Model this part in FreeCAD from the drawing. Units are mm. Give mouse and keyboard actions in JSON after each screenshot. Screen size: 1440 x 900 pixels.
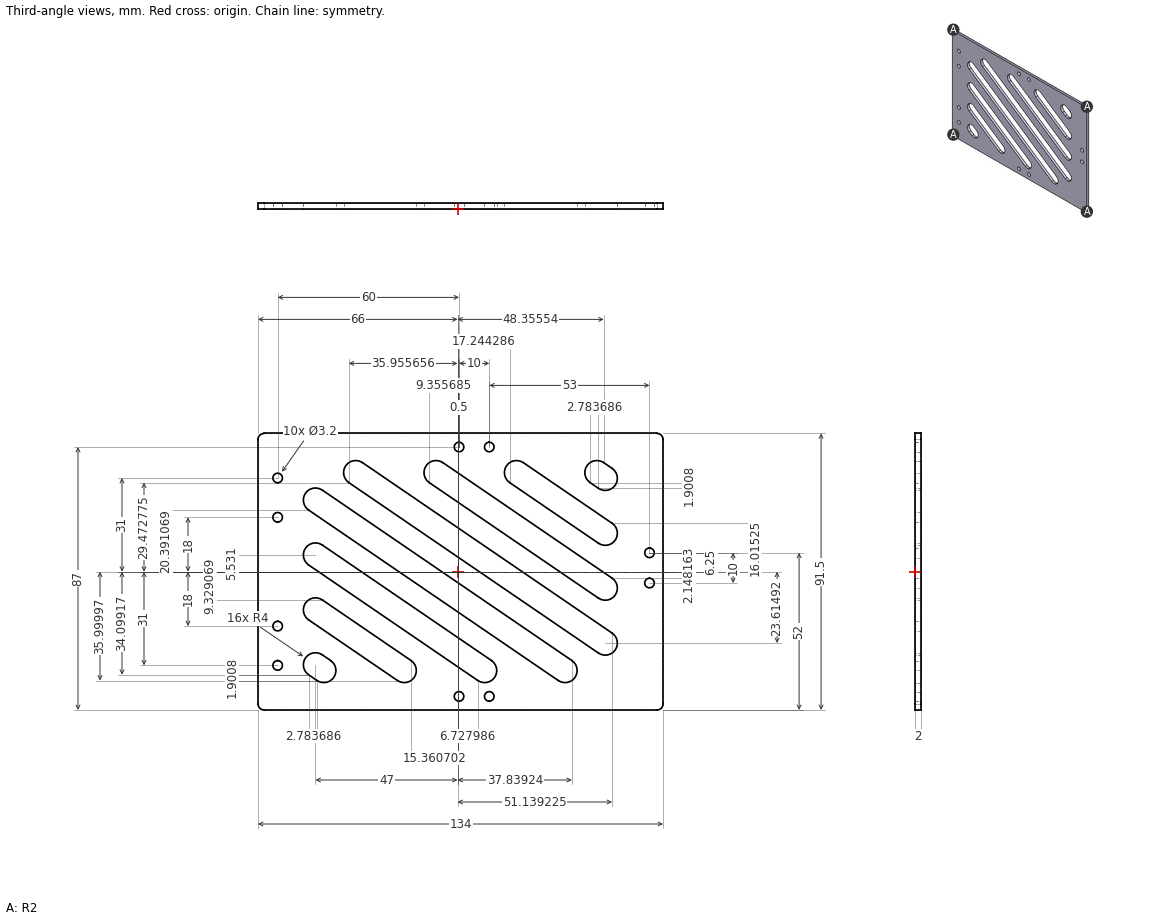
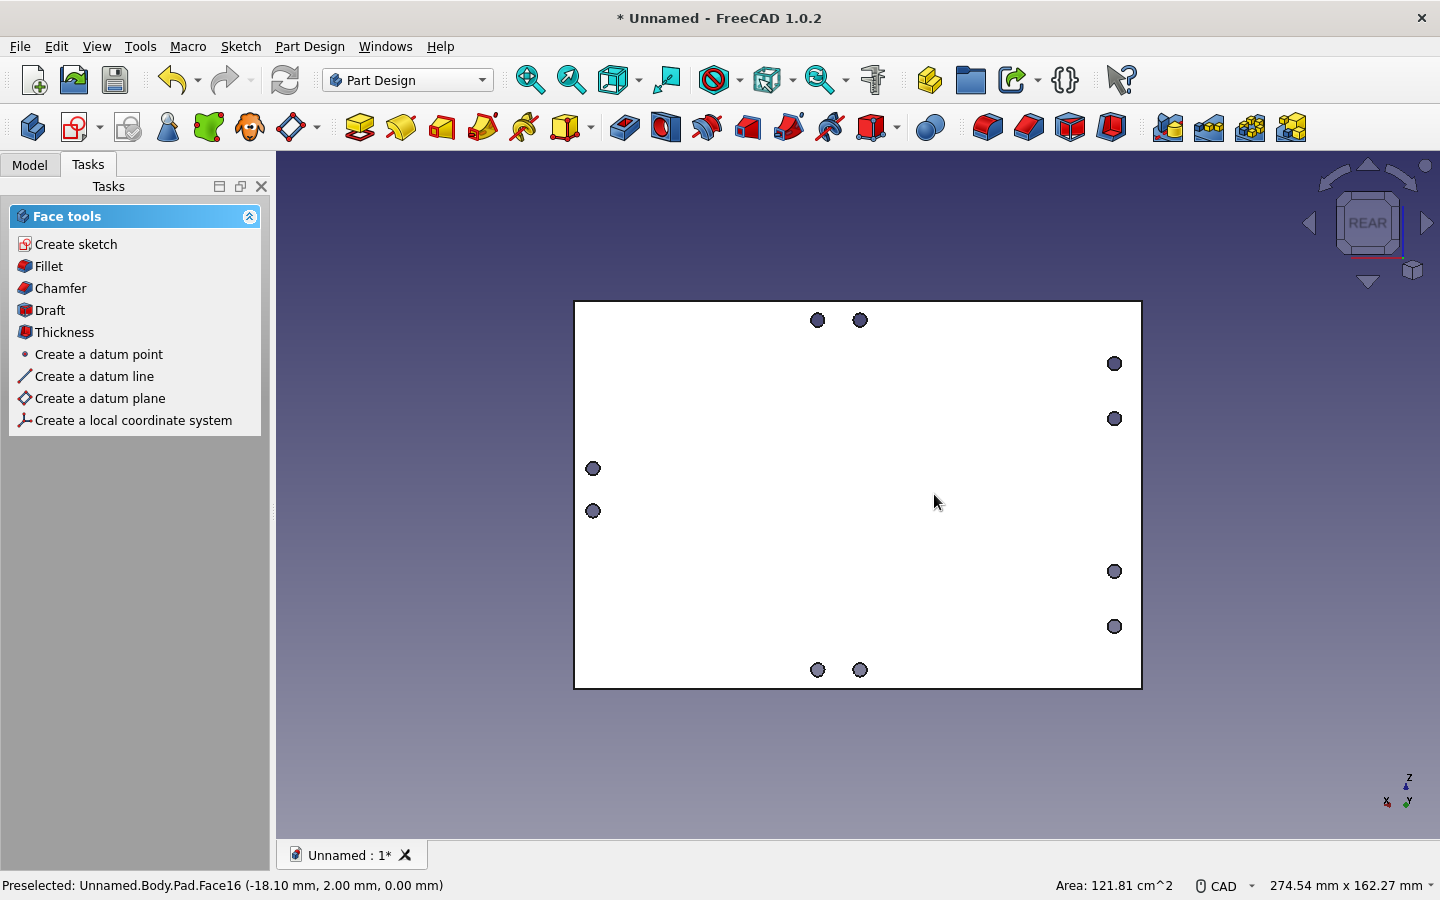
{"action": "left_click", "coordinate": [74, 128]}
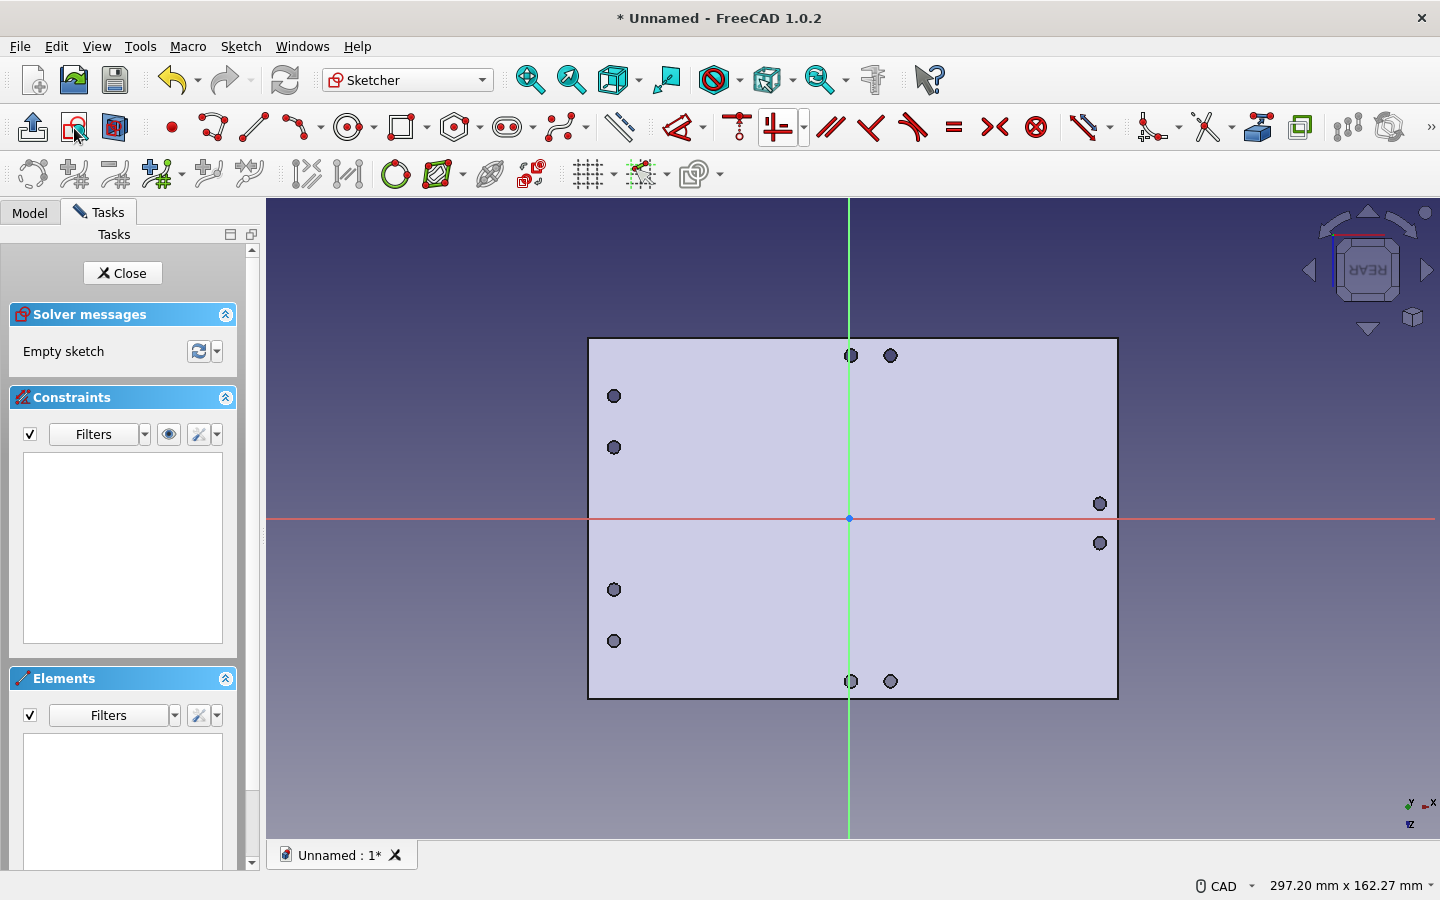
{"action": "scroll", "coordinate": [992, 519], "scroll_direction": "up", "scroll_amount": 2}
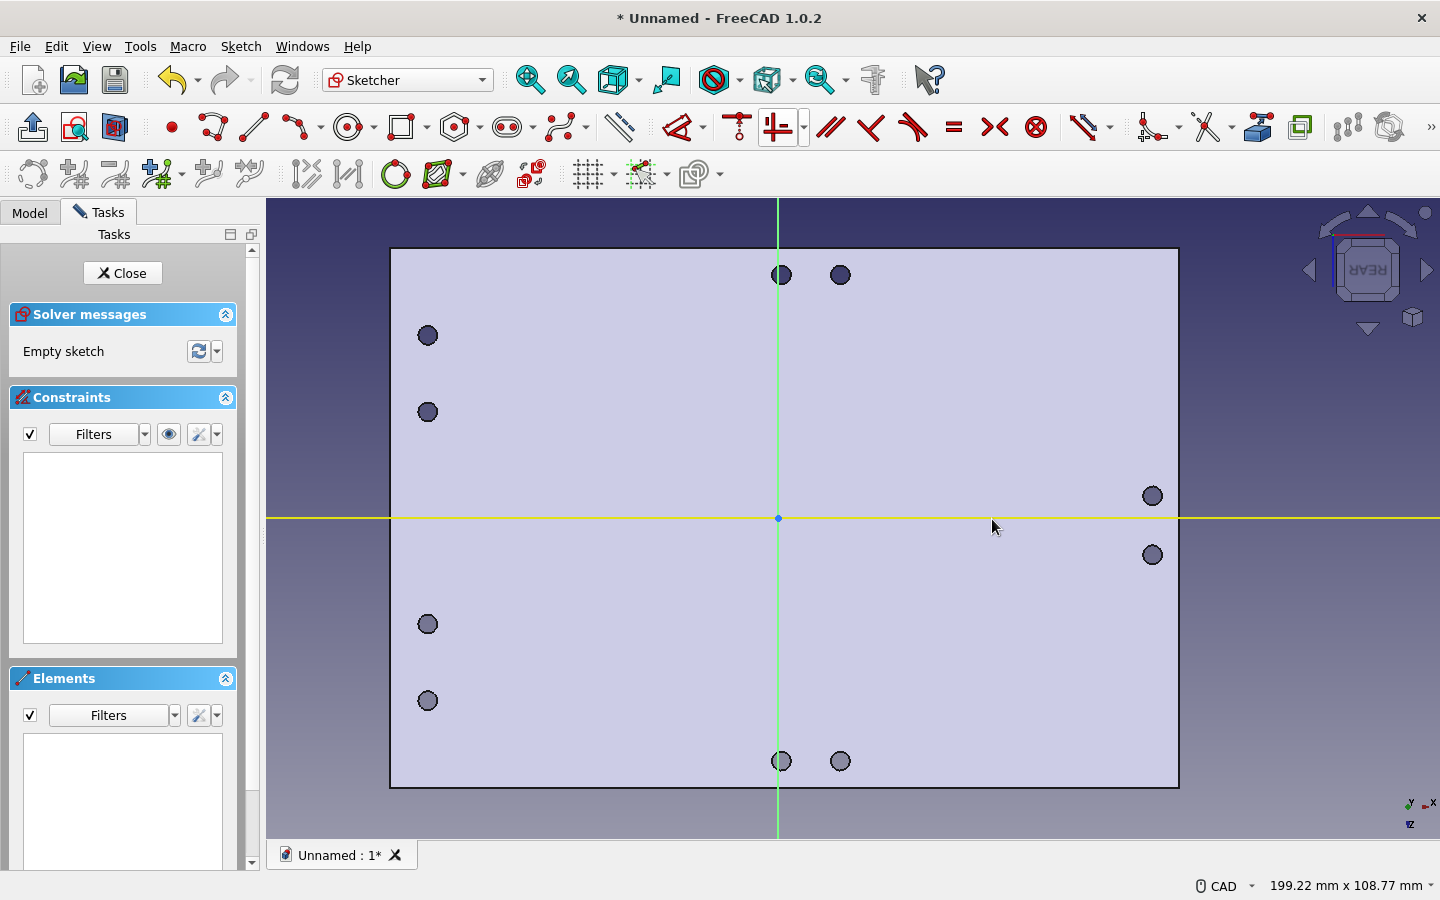
{"action": "left_click", "coordinate": [506, 128]}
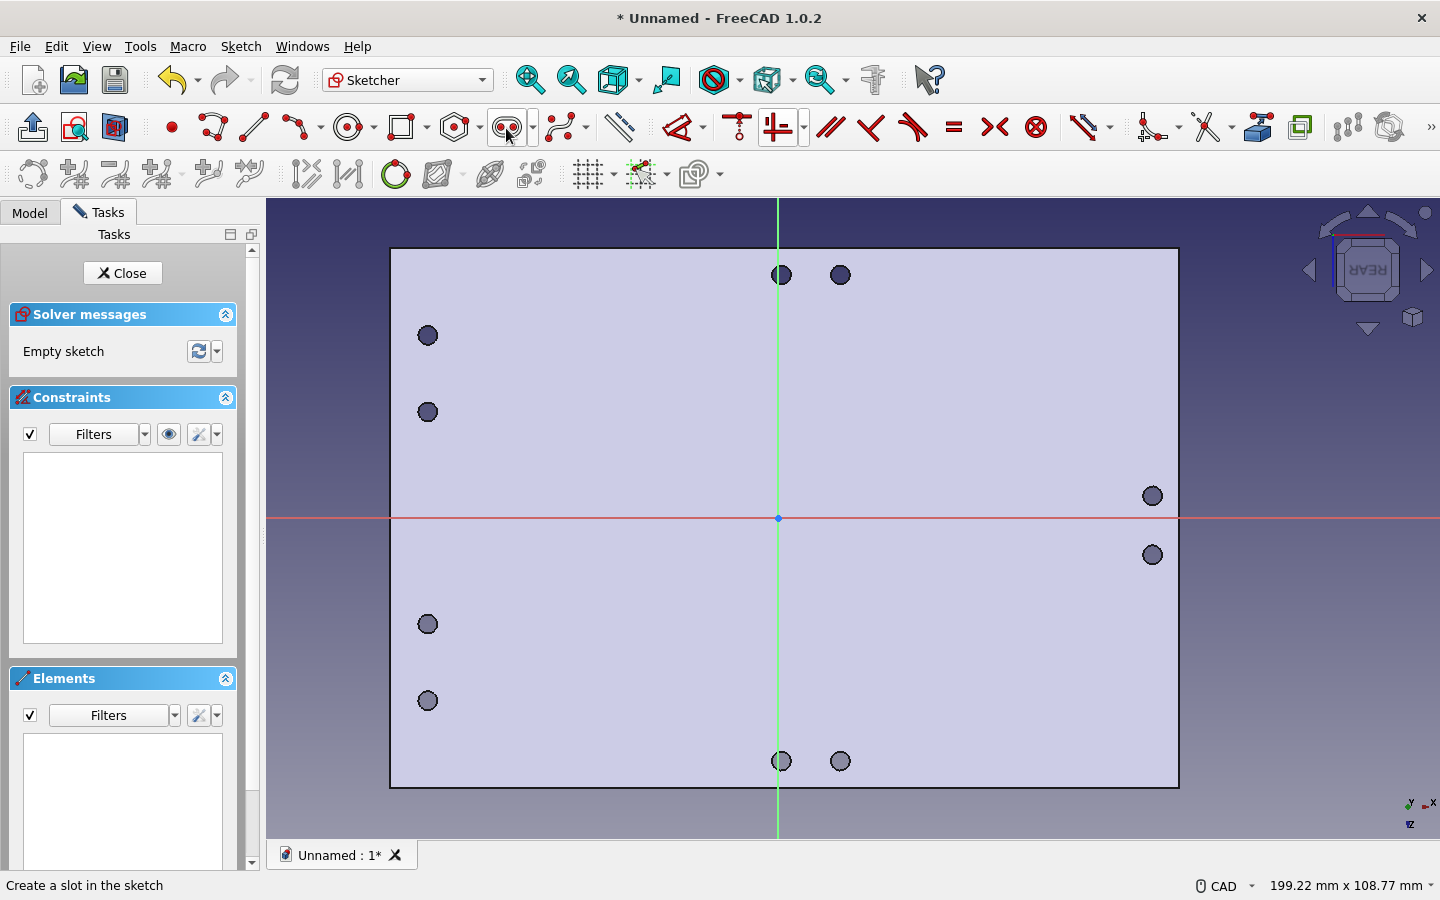
{"action": "left_click", "coordinate": [501, 337]}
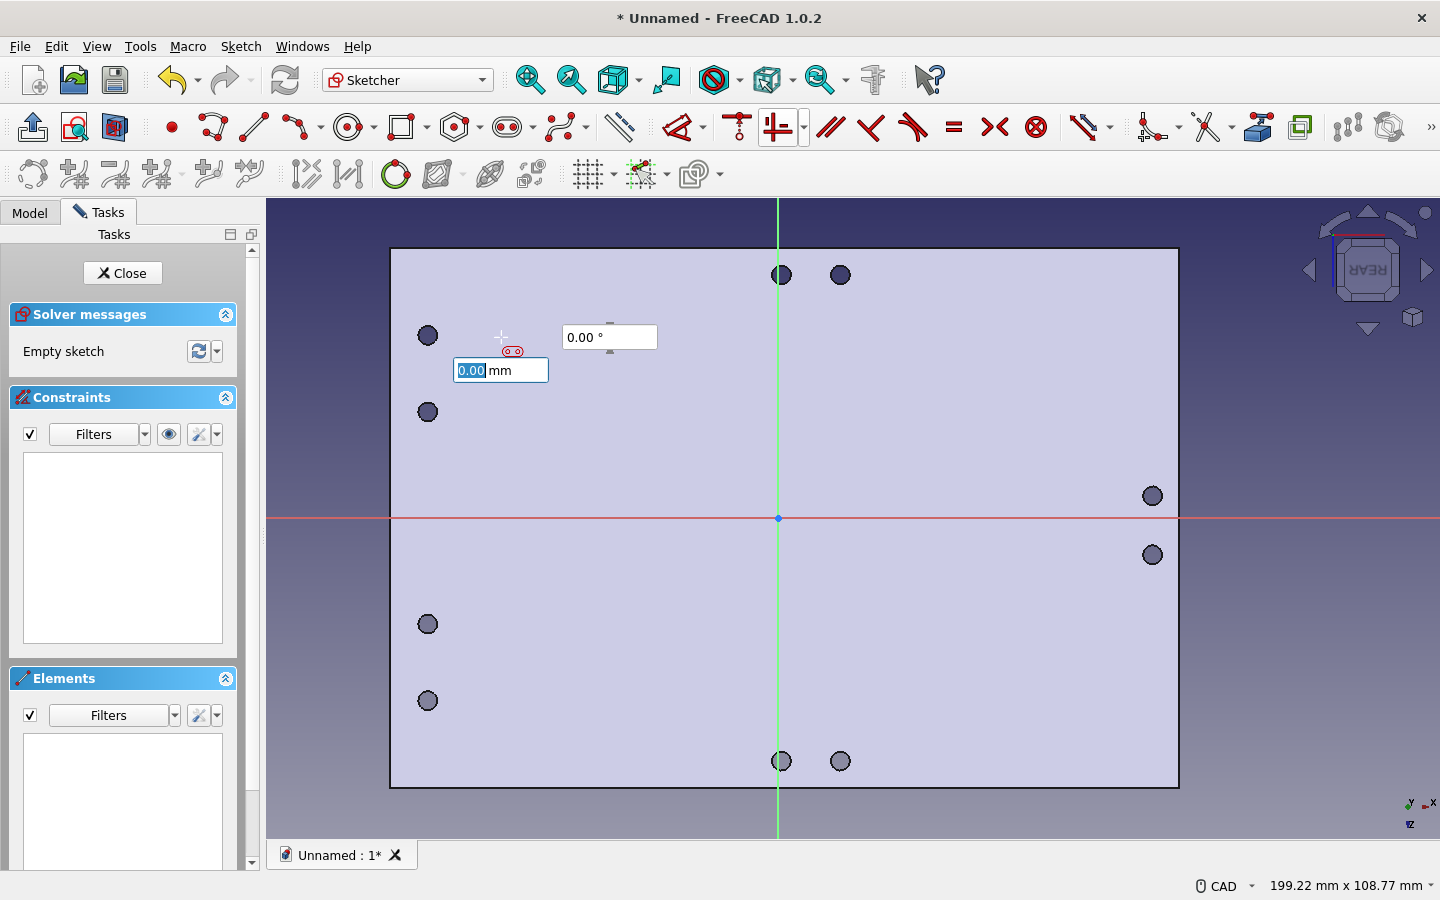
{"action": "left_click", "coordinate": [518, 325]}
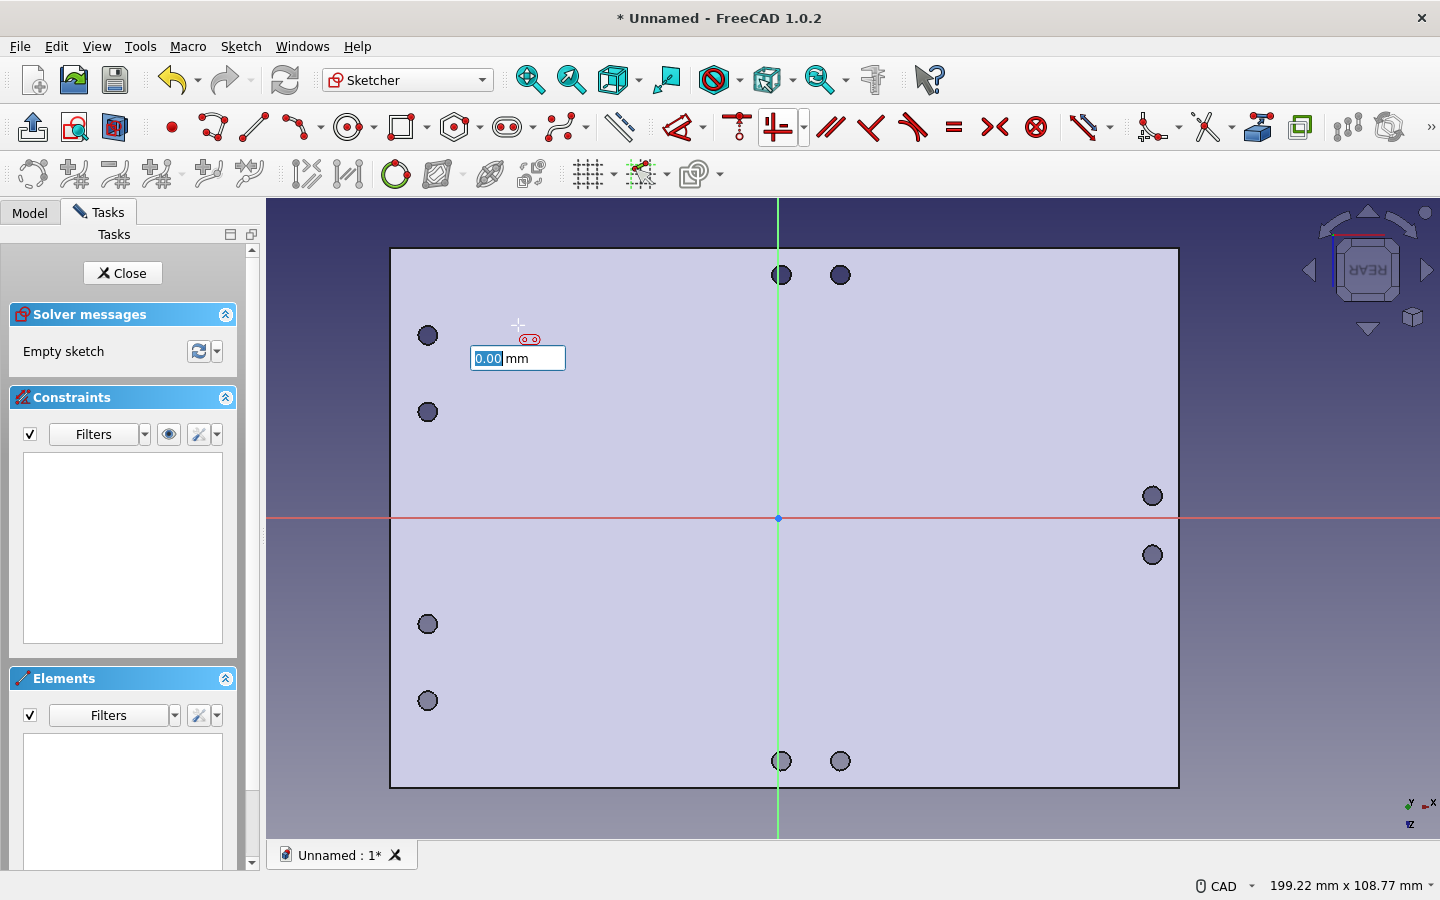
{"action": "left_click", "coordinate": [496, 311]}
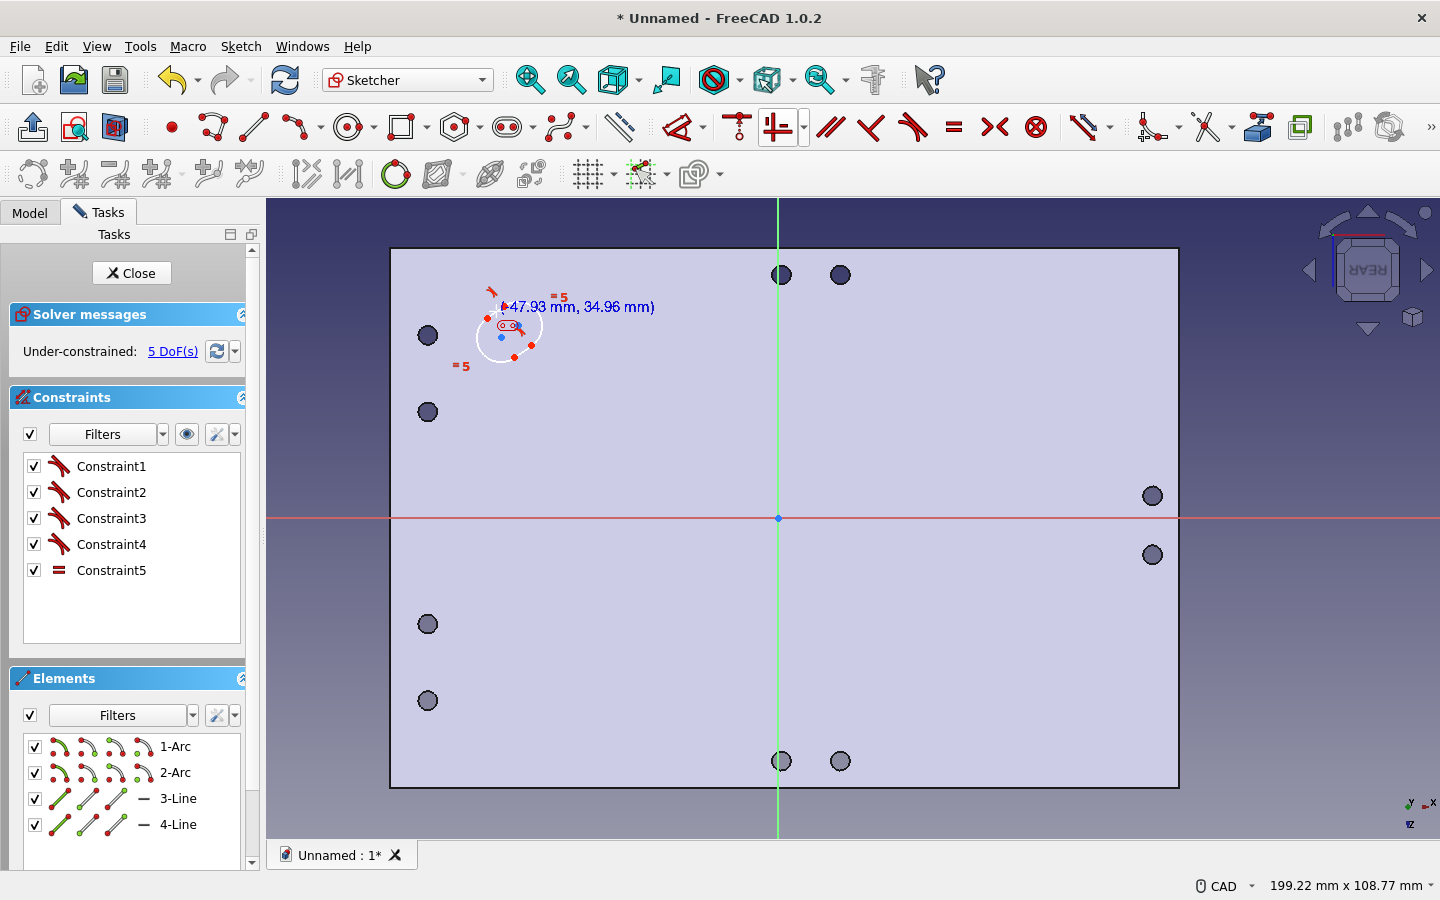
{"action": "left_click", "coordinate": [501, 444]}